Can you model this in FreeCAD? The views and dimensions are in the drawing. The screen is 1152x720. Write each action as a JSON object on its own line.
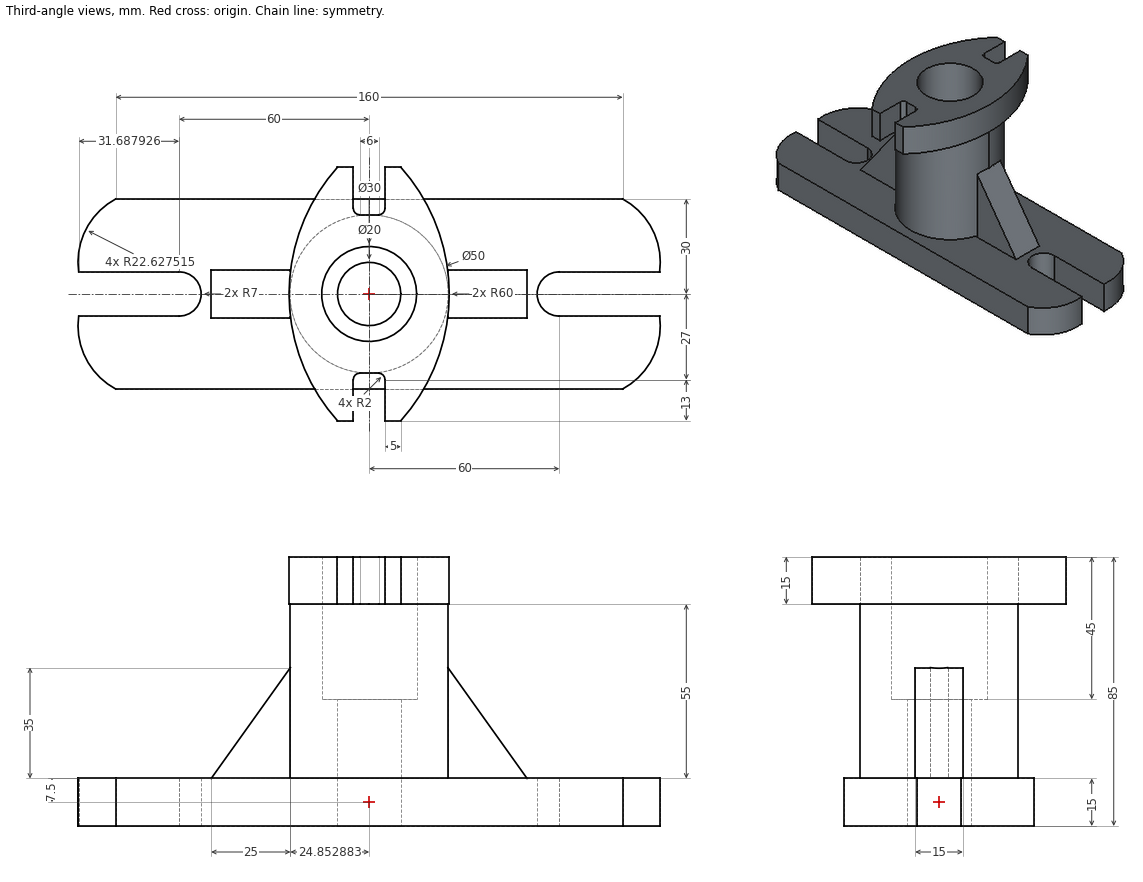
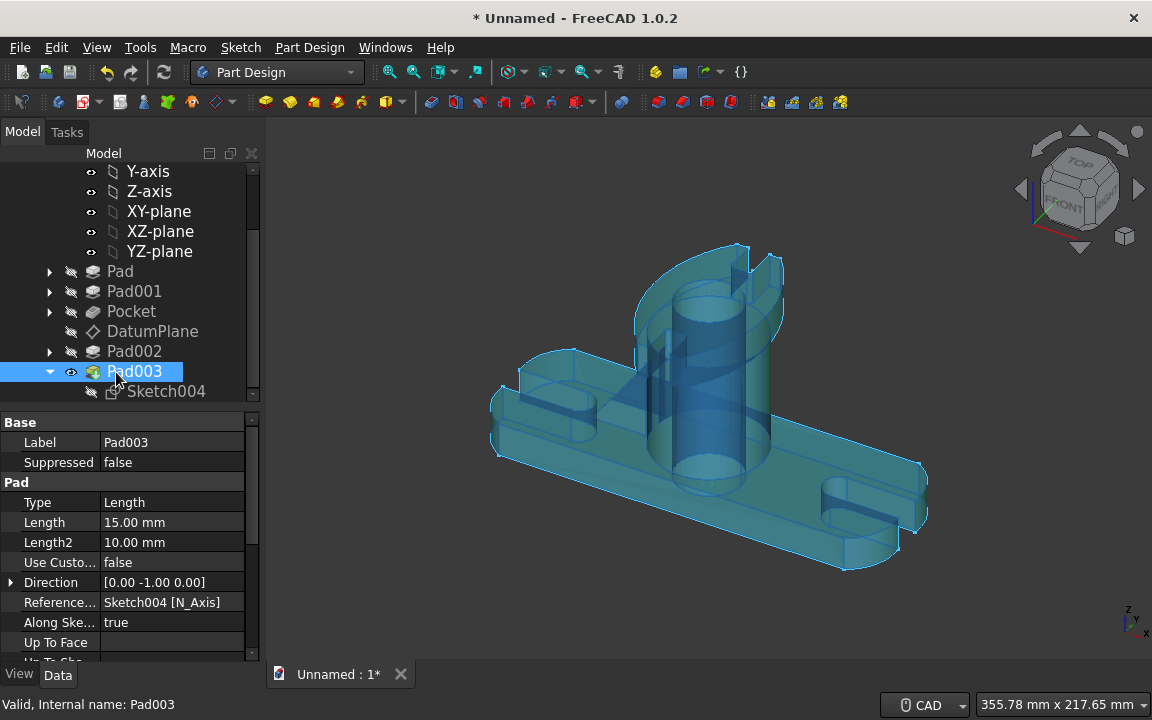
{"action": "left_click", "coordinate": [768, 102]}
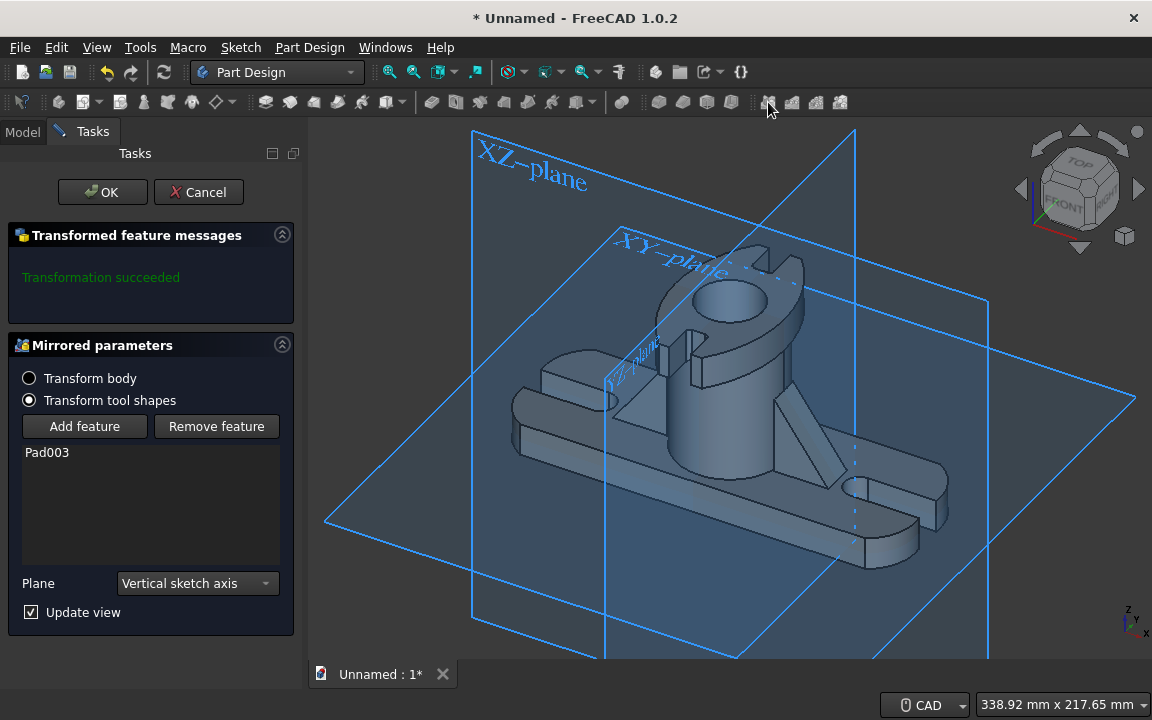
{"action": "left_click", "coordinate": [198, 584]}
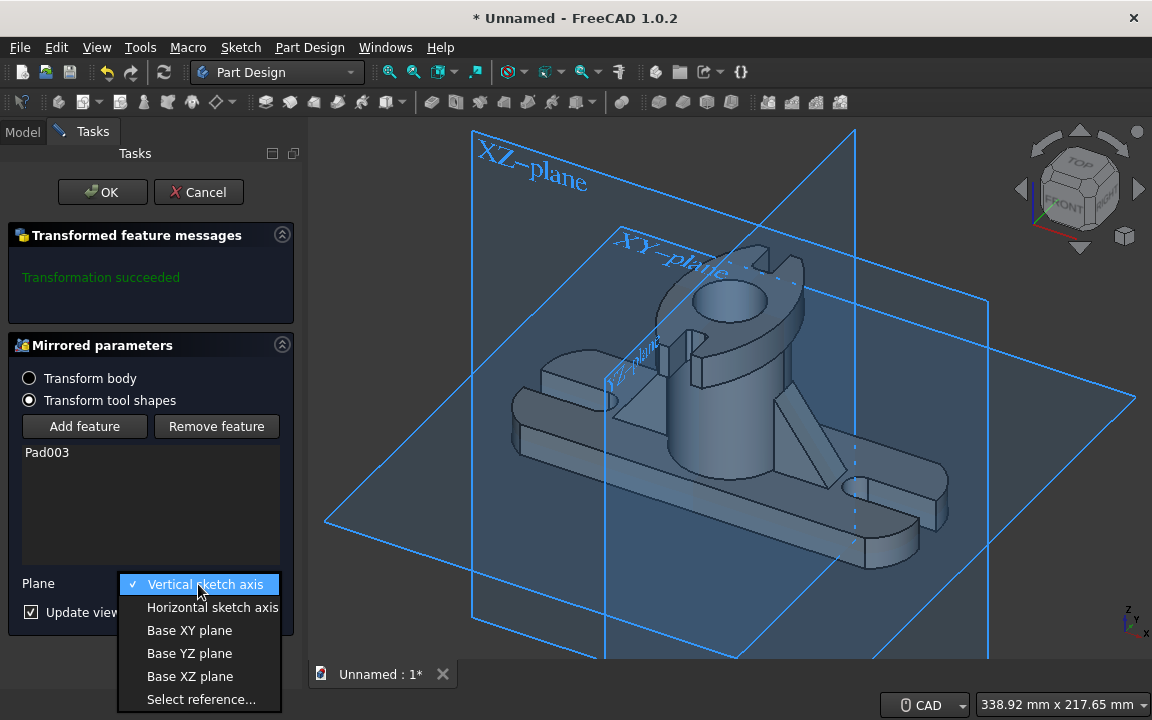
{"action": "left_click", "coordinate": [198, 654]}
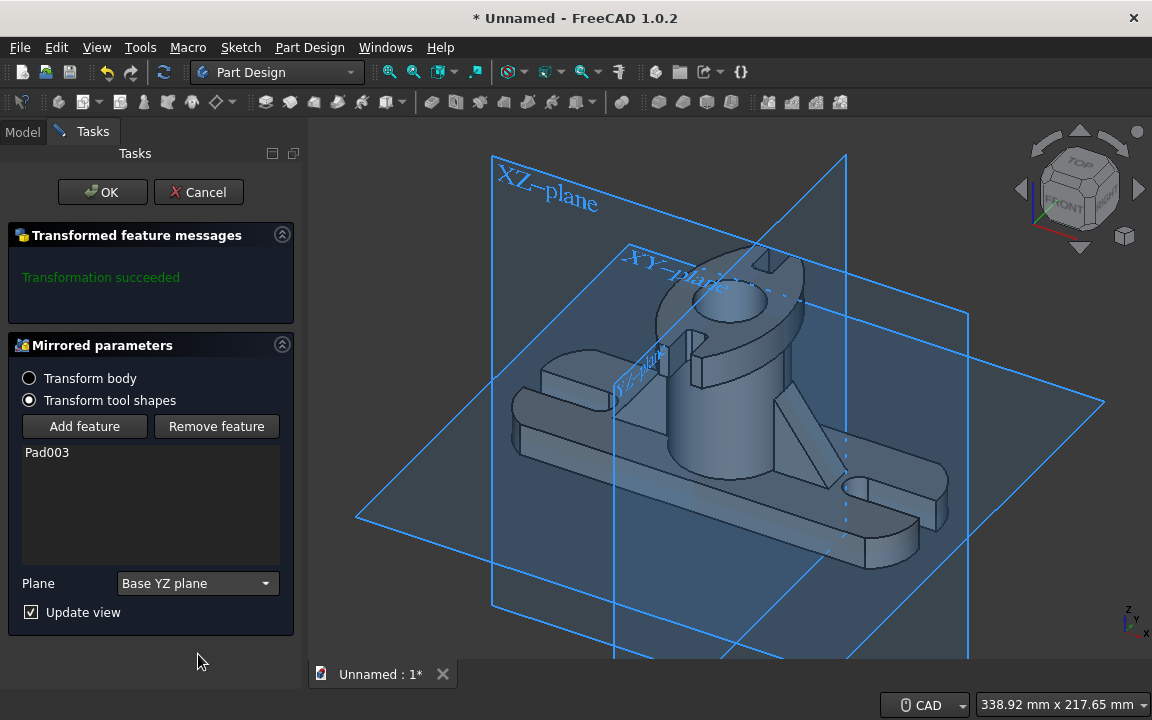
{"action": "left_click", "coordinate": [103, 192]}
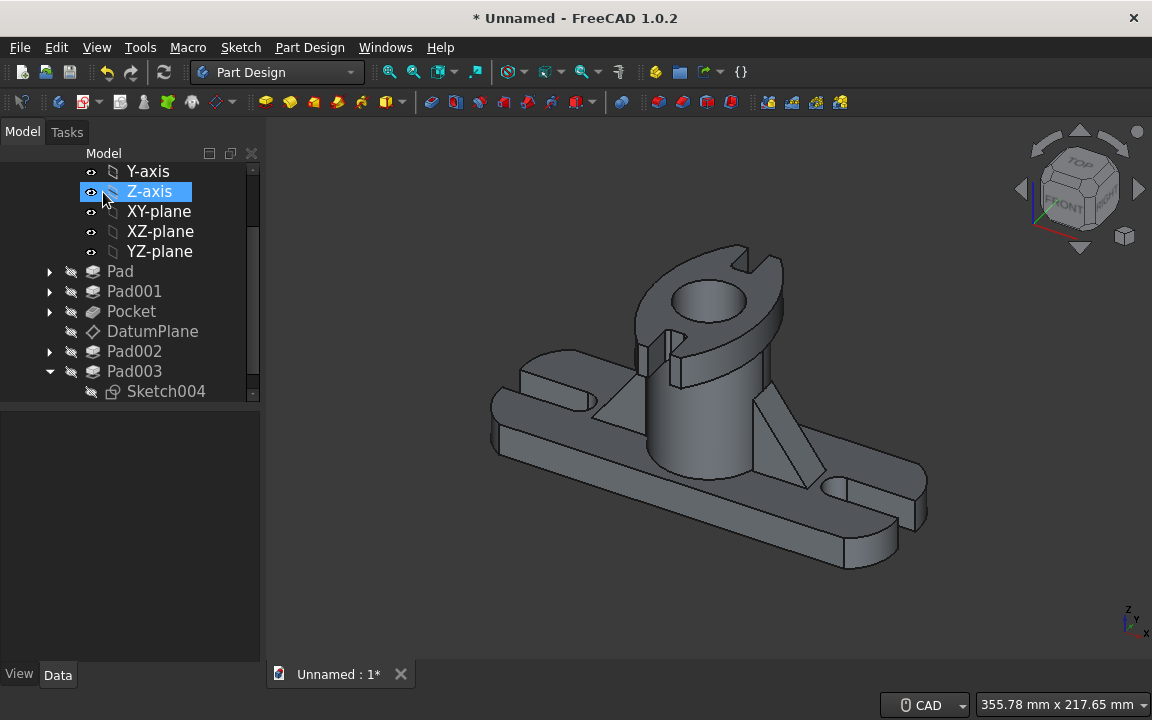
{"action": "left_click", "coordinate": [706, 262]}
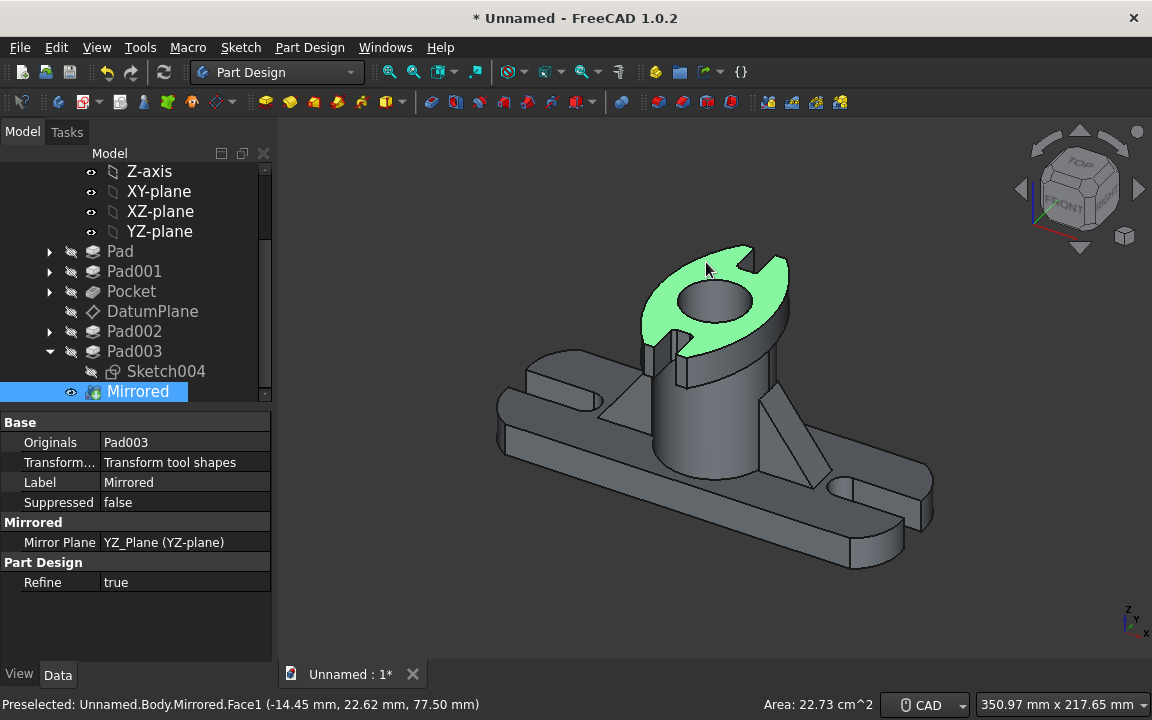
{"action": "left_click", "coordinate": [84, 102]}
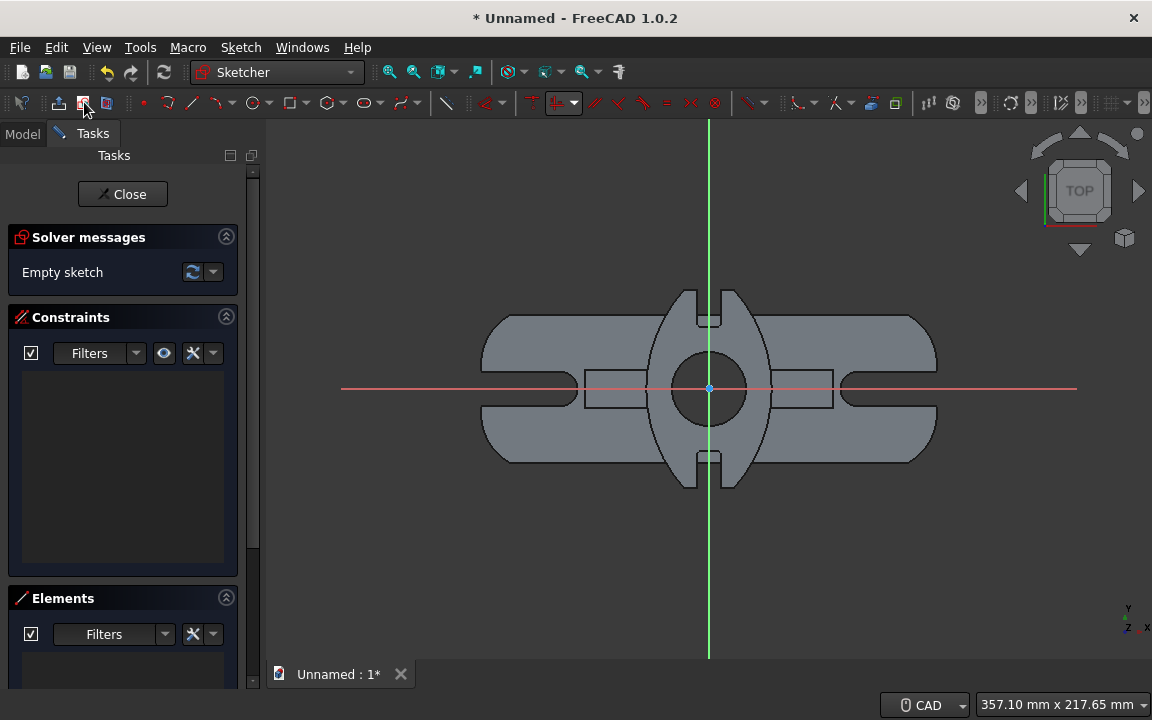
{"action": "scroll", "coordinate": [726, 389], "scroll_direction": "up", "scroll_amount": 8}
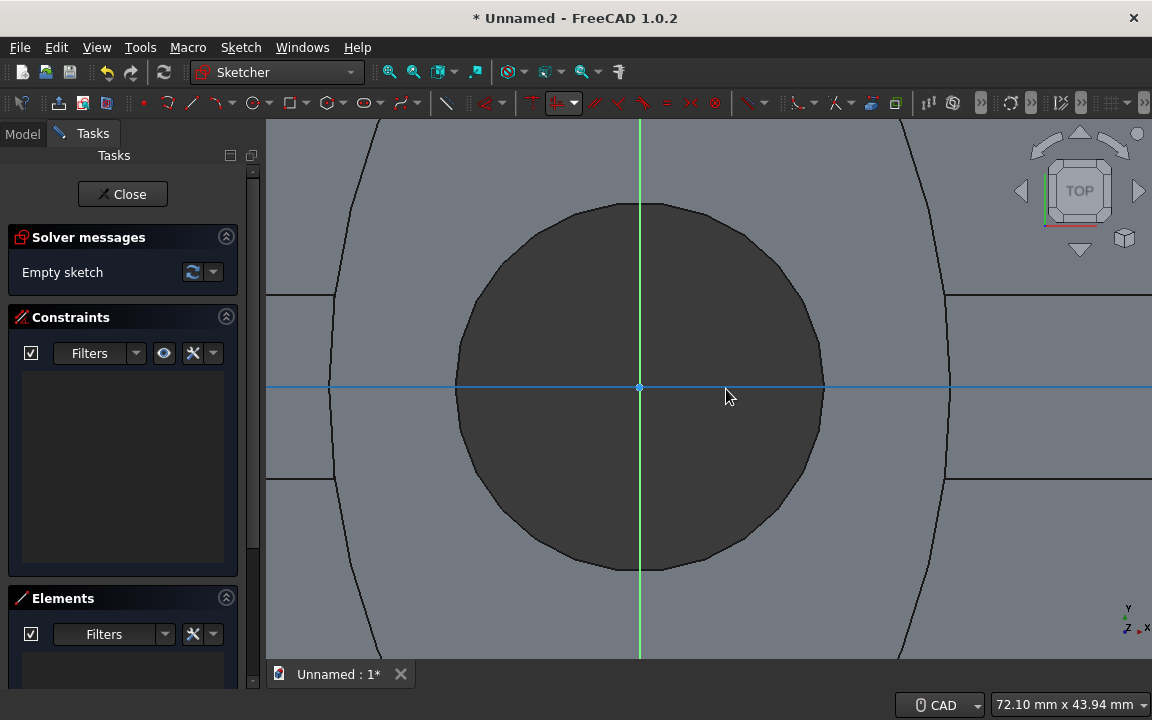
{"action": "key", "text": "g c"}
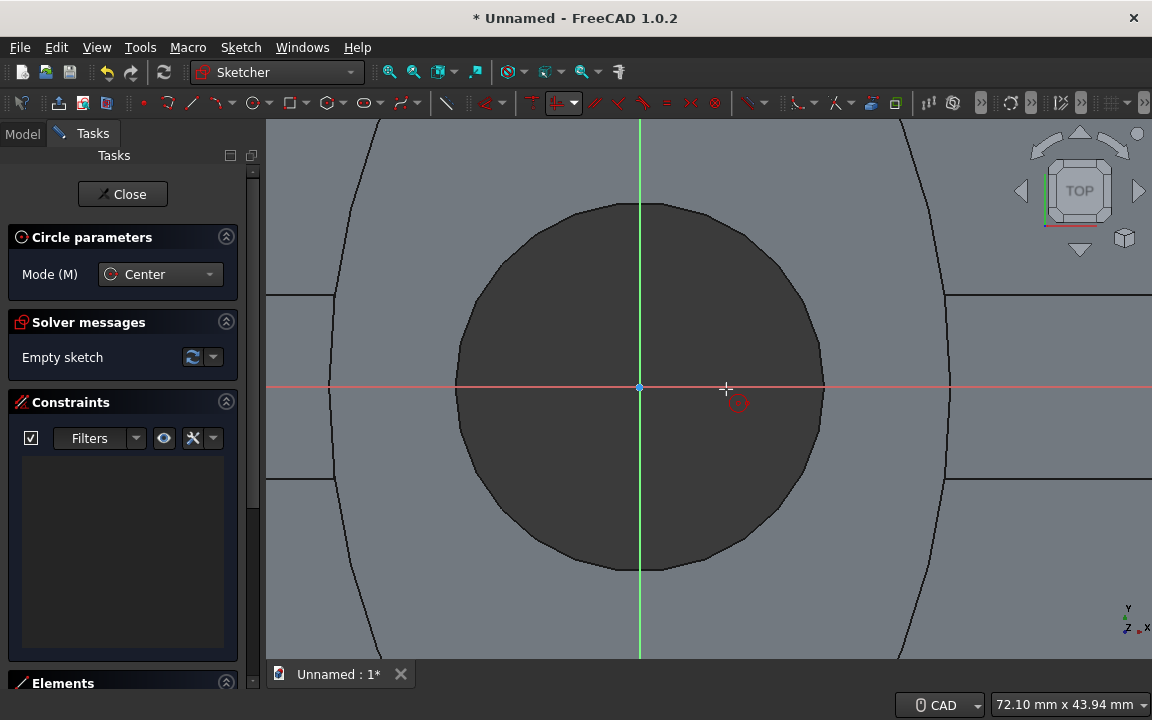
{"action": "left_click", "coordinate": [640, 387]}
{"action": "mouse_move", "coordinate": [770, 257]}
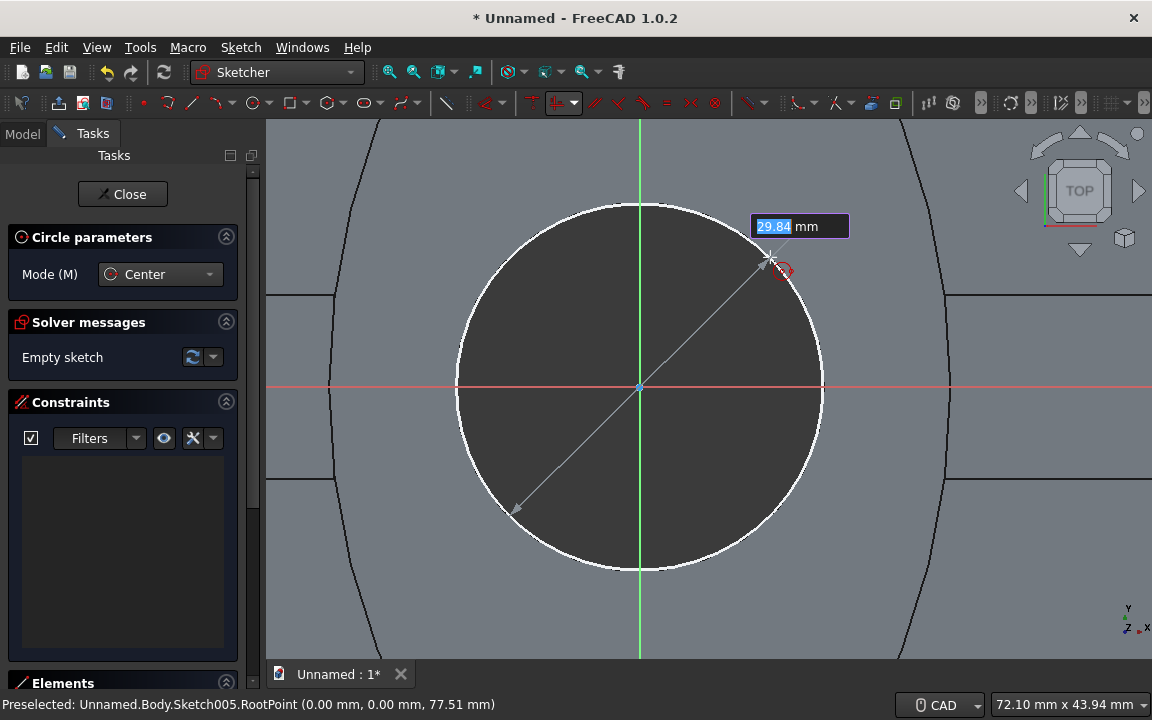
{"action": "type", "text": "30"}
{"action": "key", "text": "Return"}
{"action": "key", "text": "Escape"}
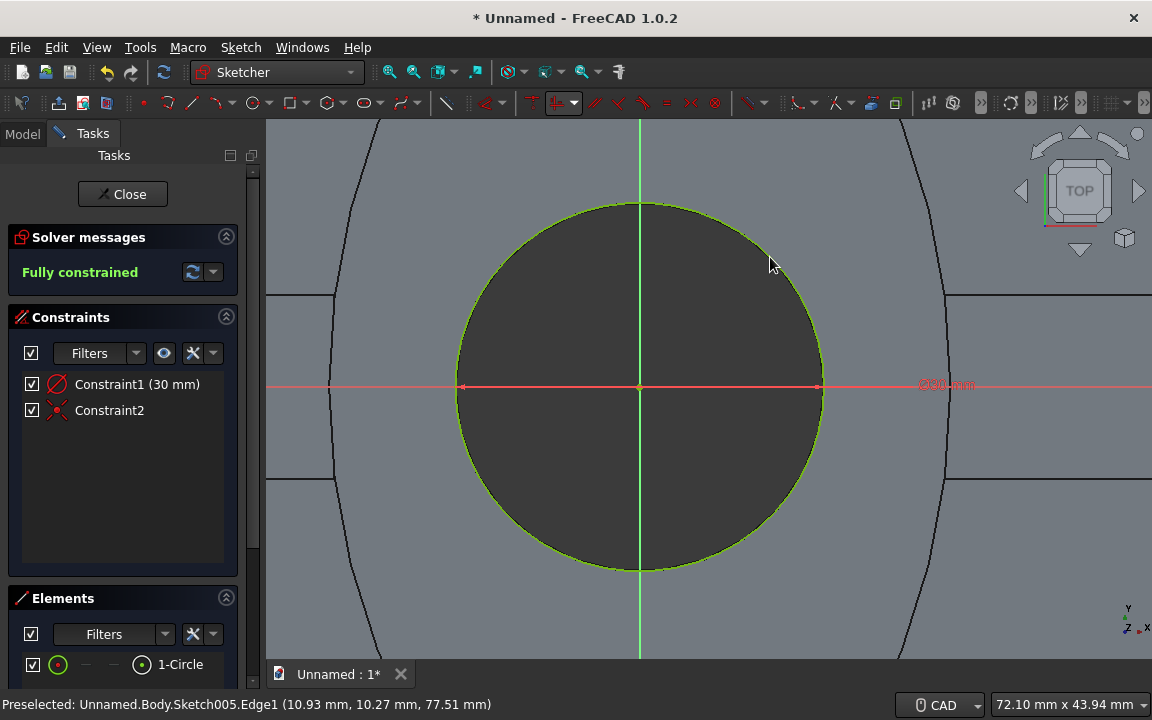
{"action": "left_click", "coordinate": [123, 194]}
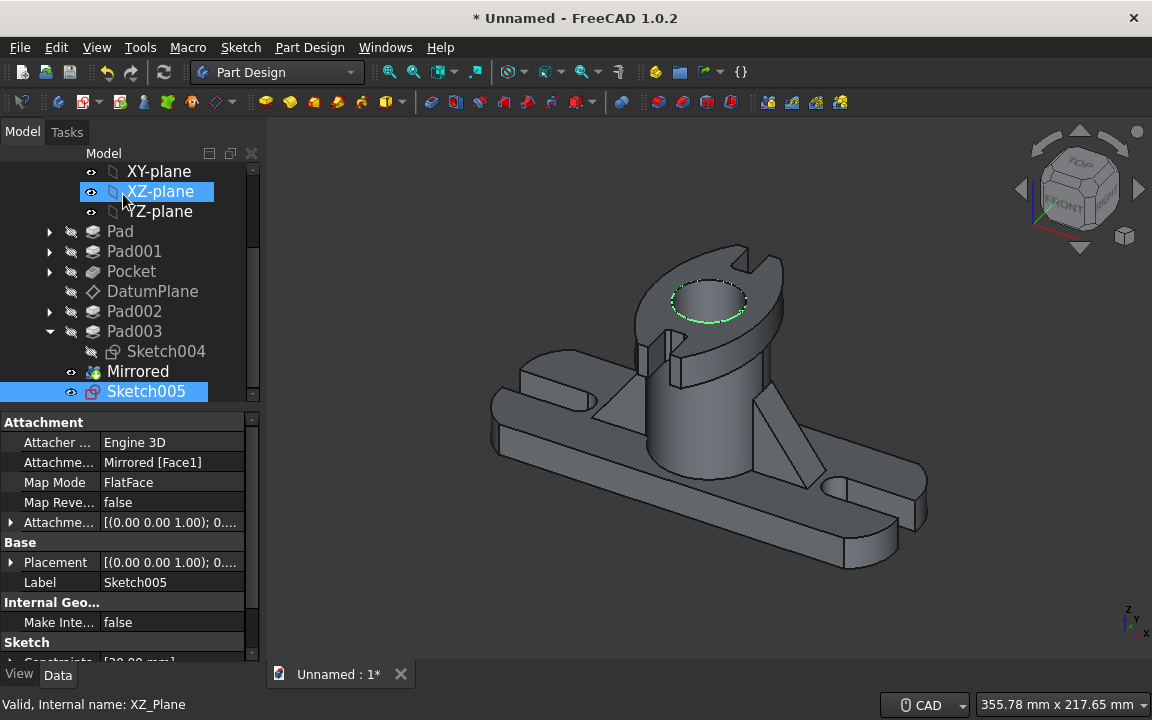
{"action": "left_click", "coordinate": [266, 102]}